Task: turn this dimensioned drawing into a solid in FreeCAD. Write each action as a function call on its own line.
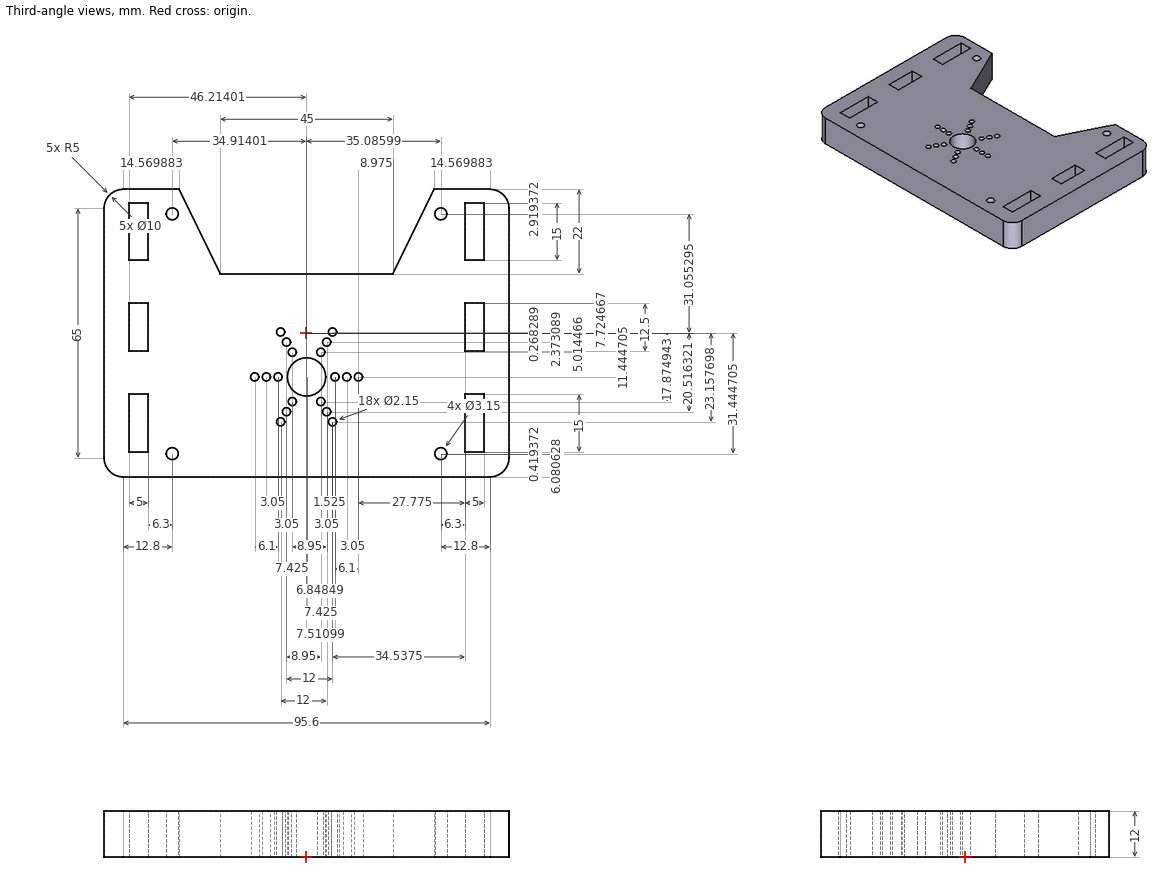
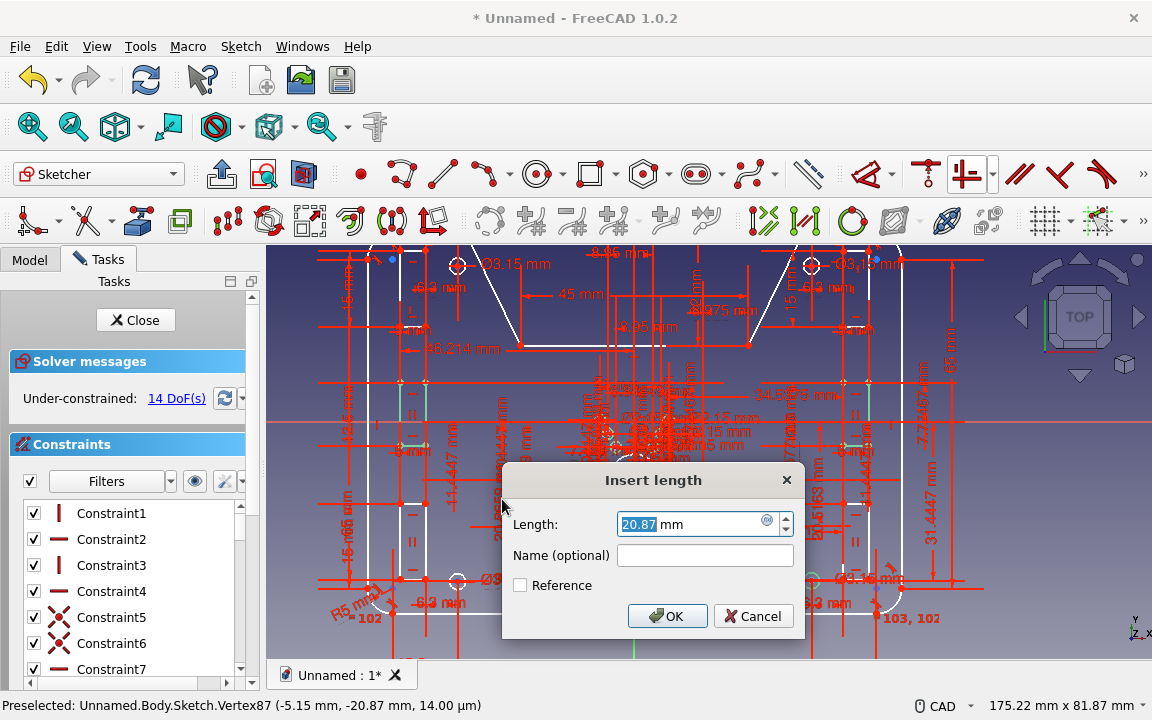
text(20.516321)
key(Return)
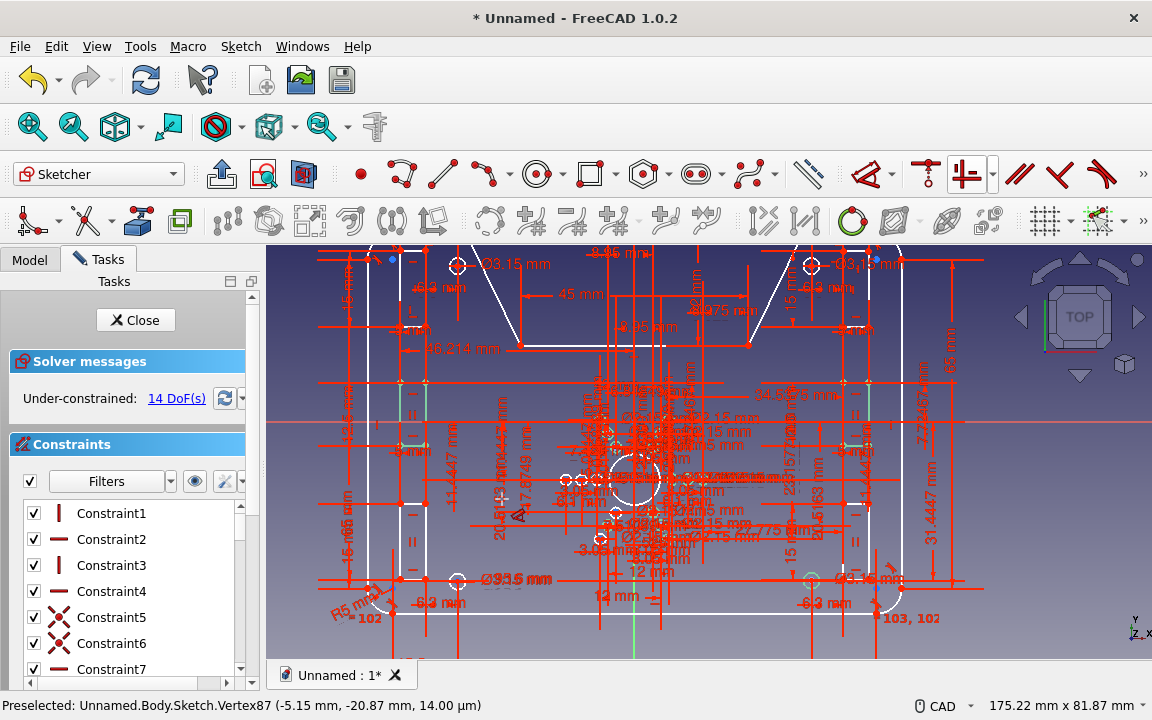
click(600, 539)
click(494, 522)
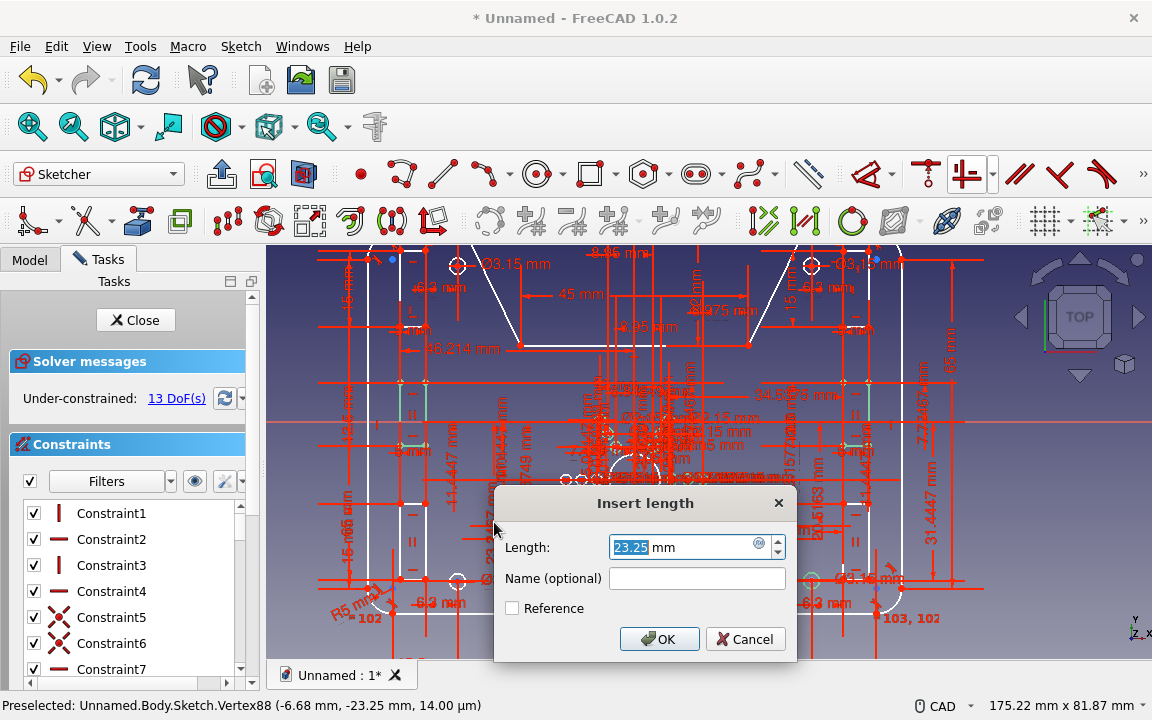
text(23.157698)
key(Return)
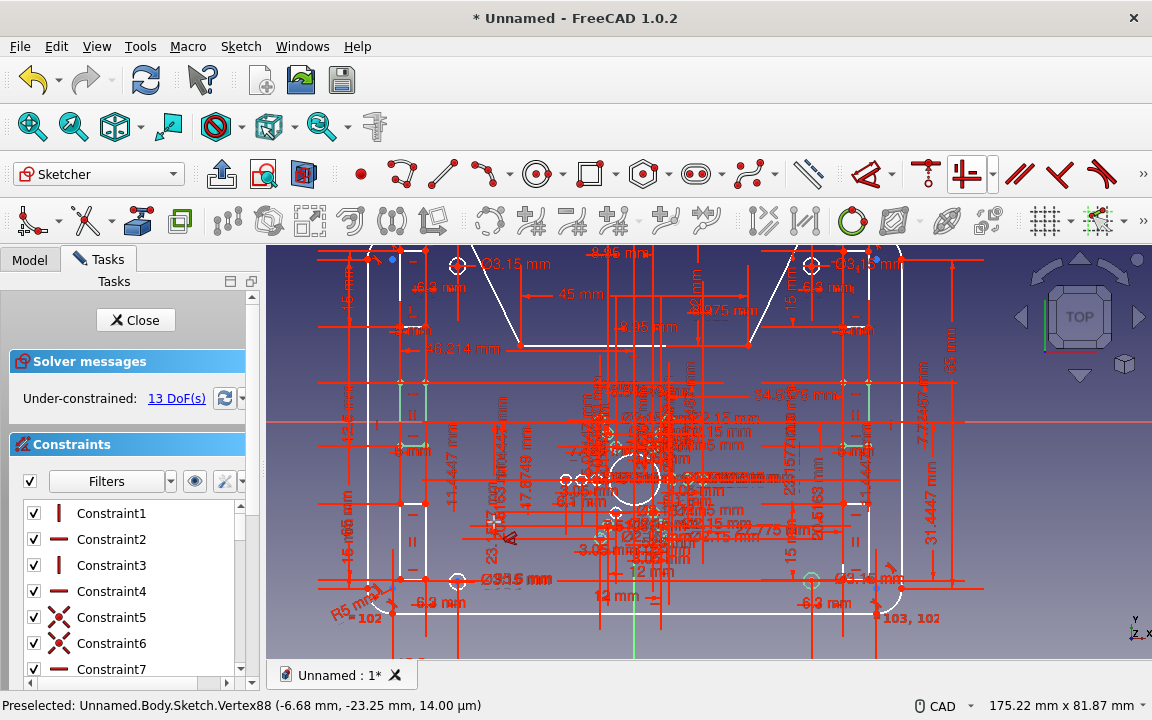
click(616, 513)
click(582, 467)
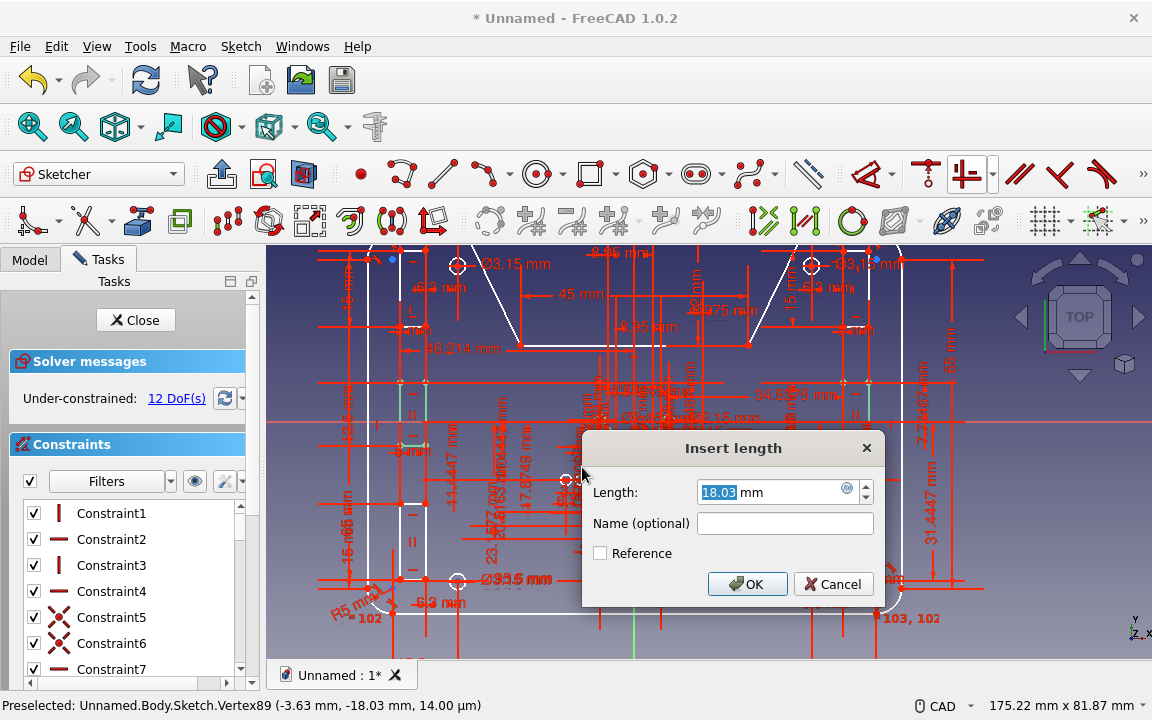
text(17.874943)
key(Return)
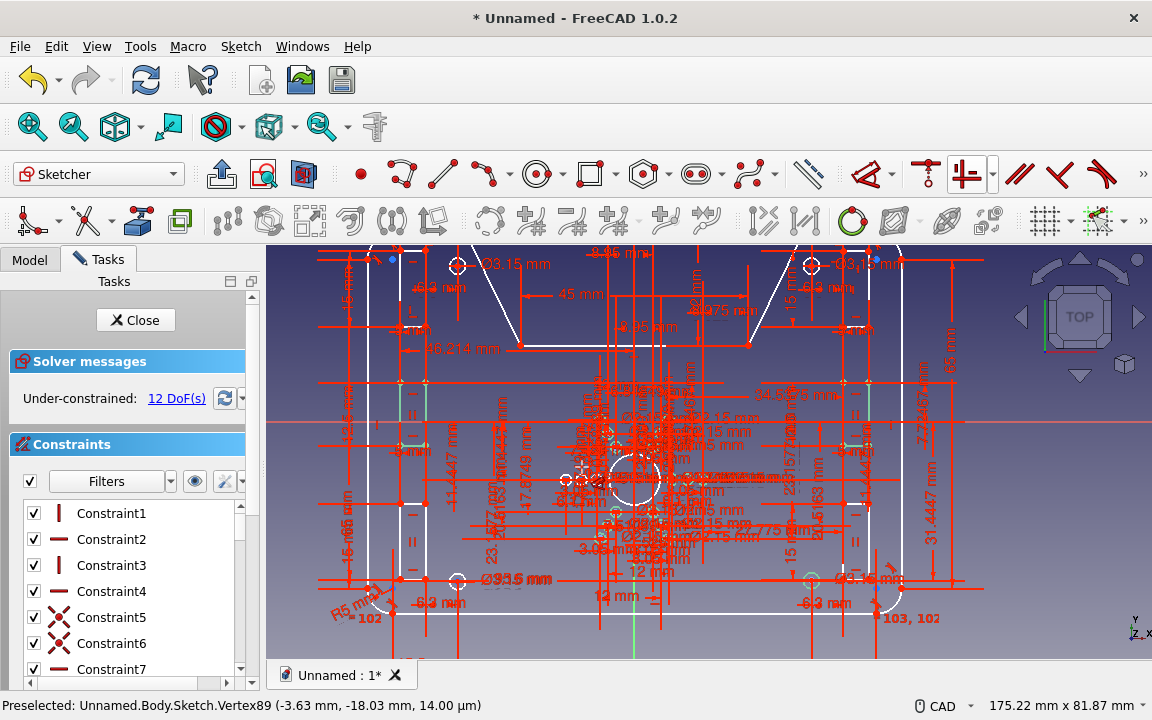
click(458, 582)
click(352, 465)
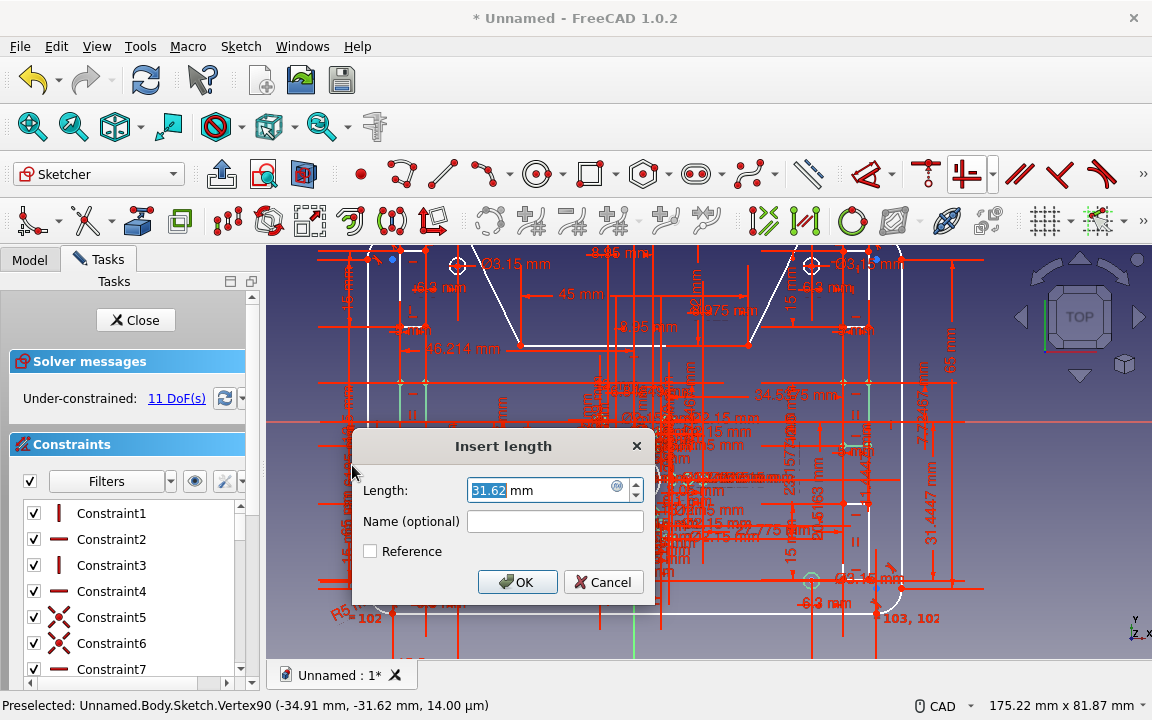
text(31.444705)
key(Return)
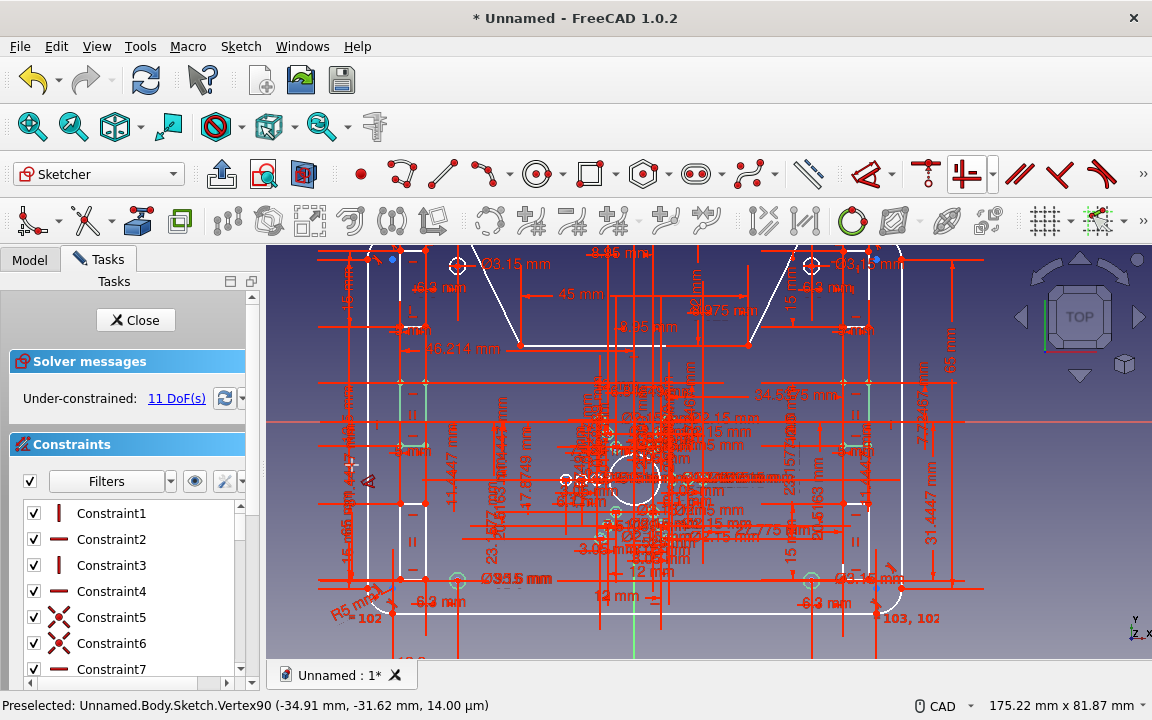
click(635, 480)
click(552, 451)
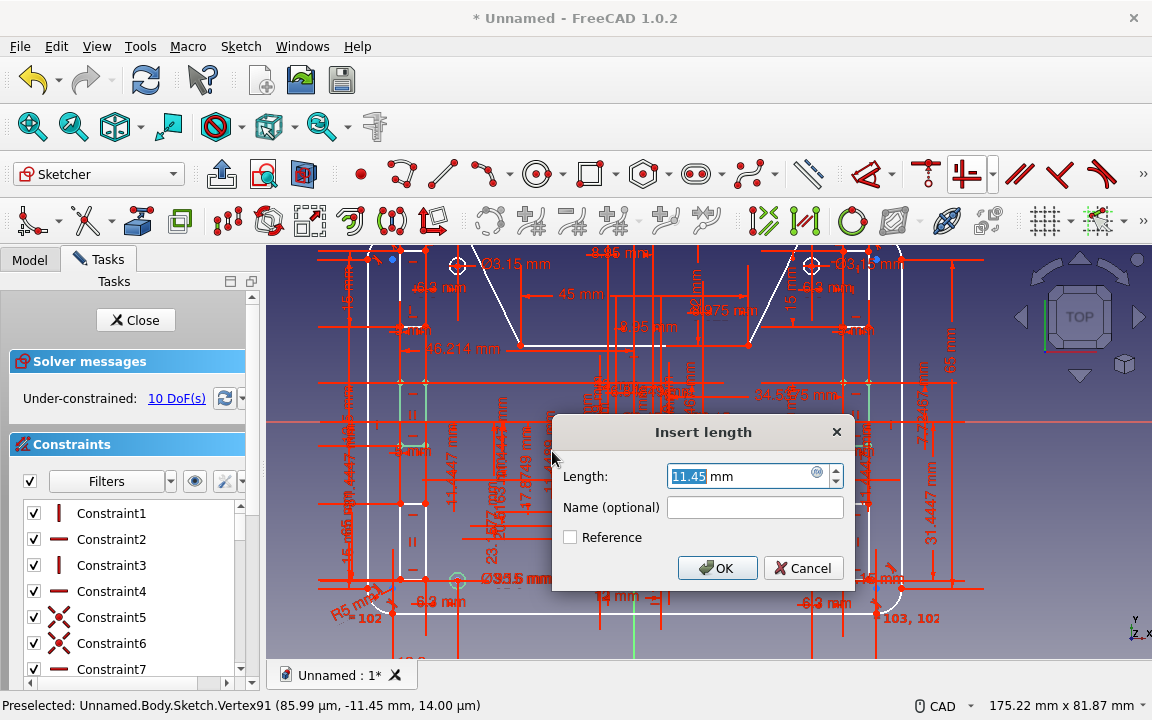
text(11.444705)
key(Return)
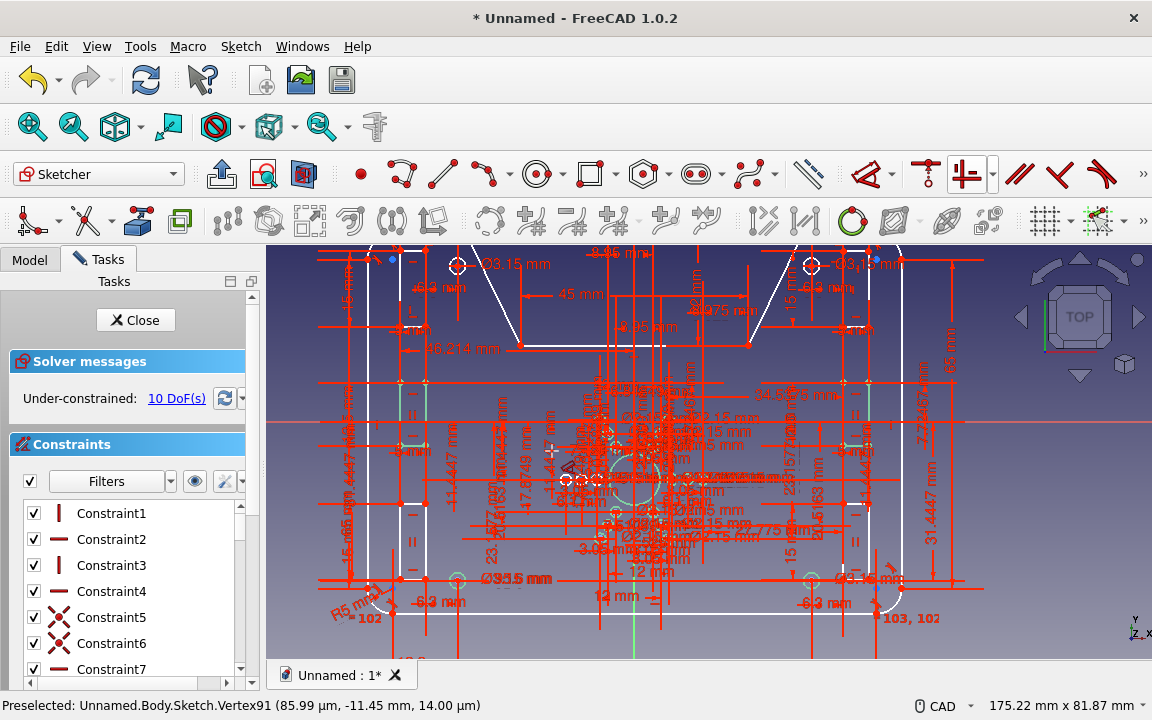
click(597, 480)
click(515, 451)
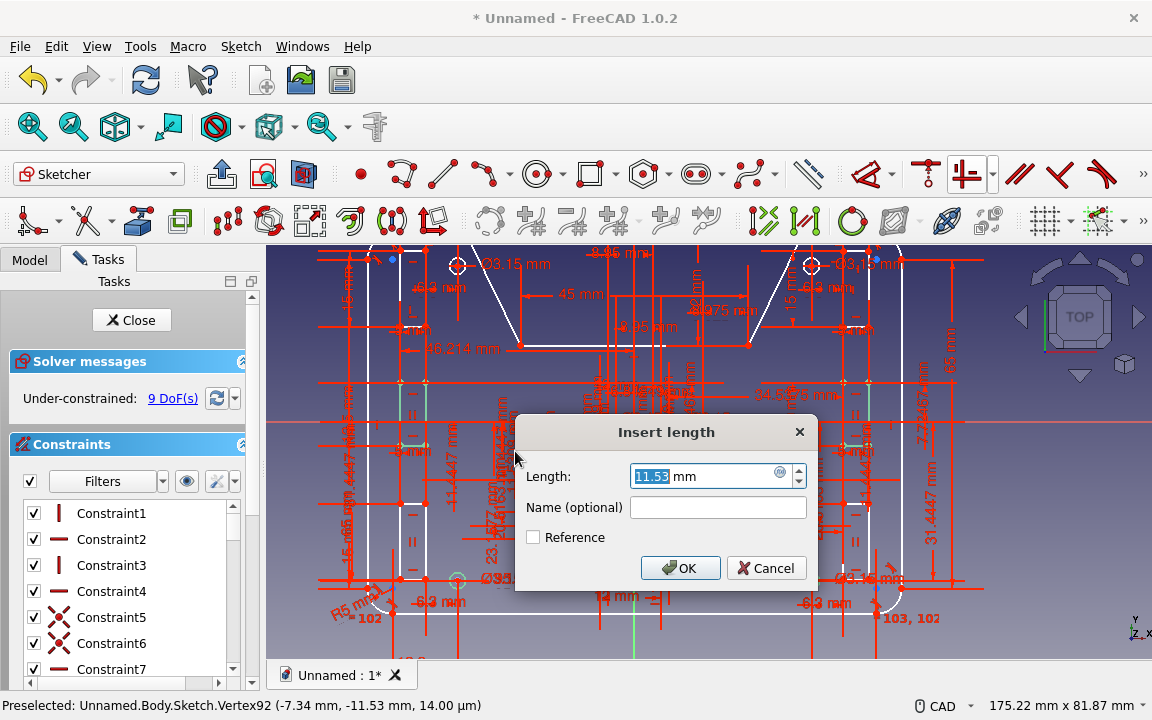
text(11.444705)
key(Return)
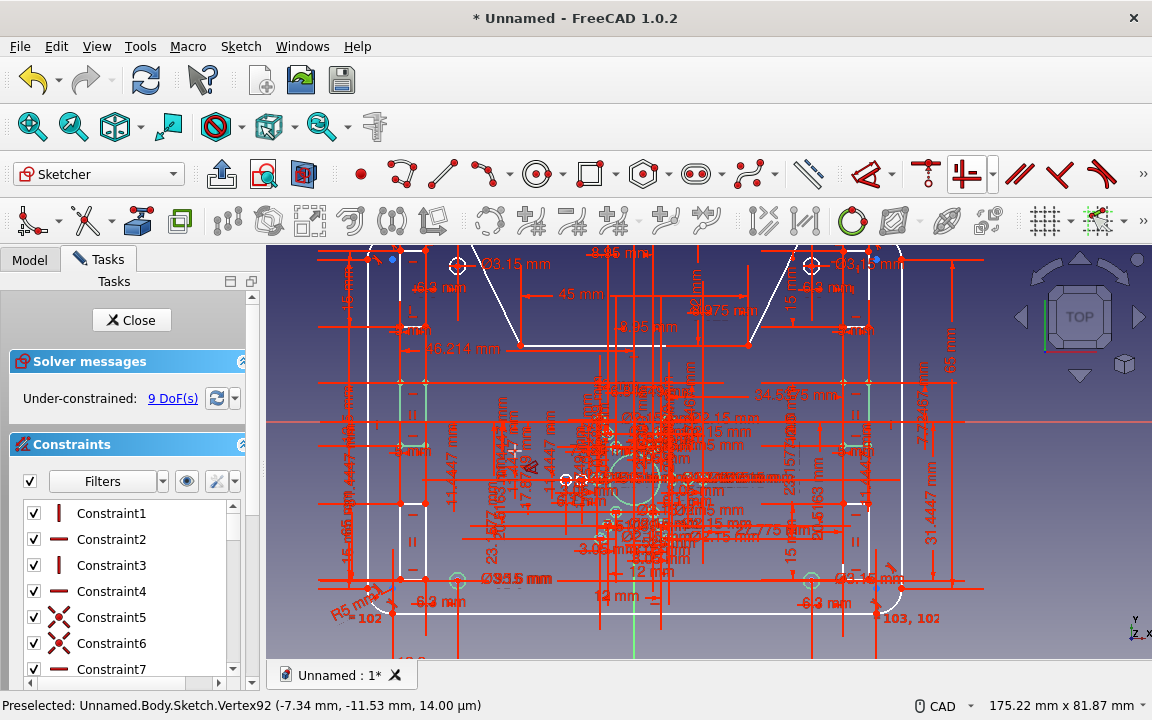
click(582, 480)
click(548, 437)